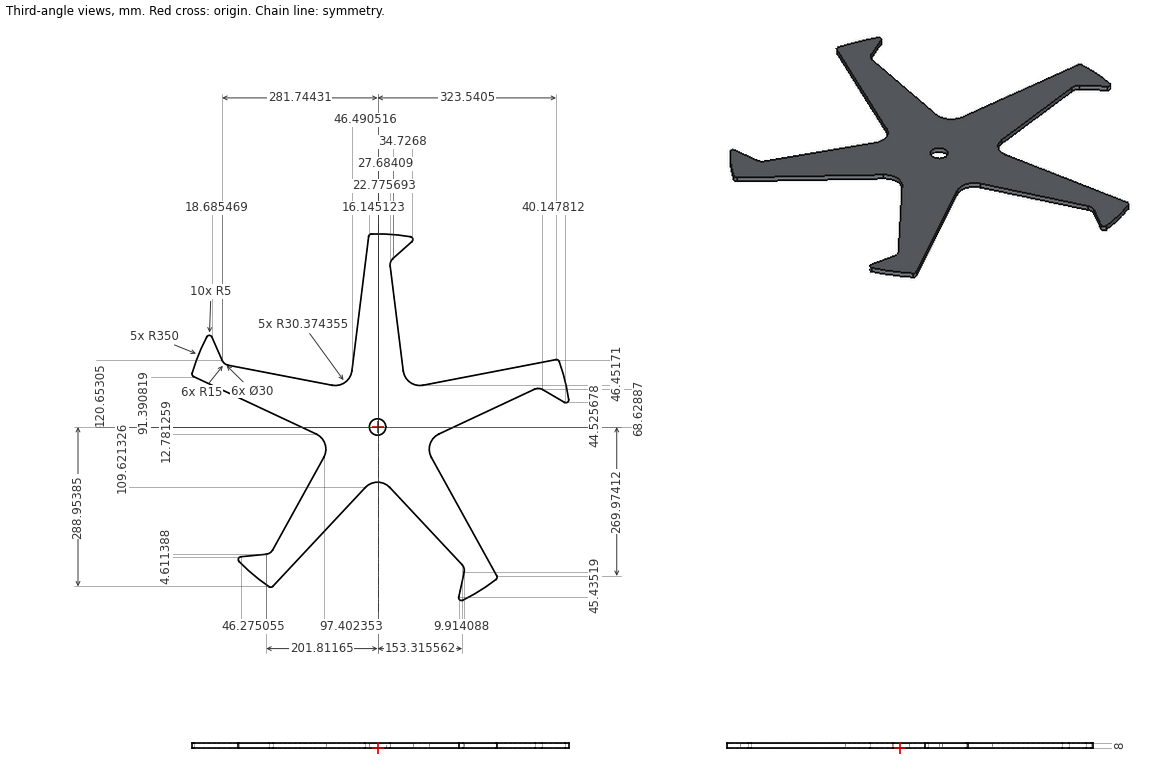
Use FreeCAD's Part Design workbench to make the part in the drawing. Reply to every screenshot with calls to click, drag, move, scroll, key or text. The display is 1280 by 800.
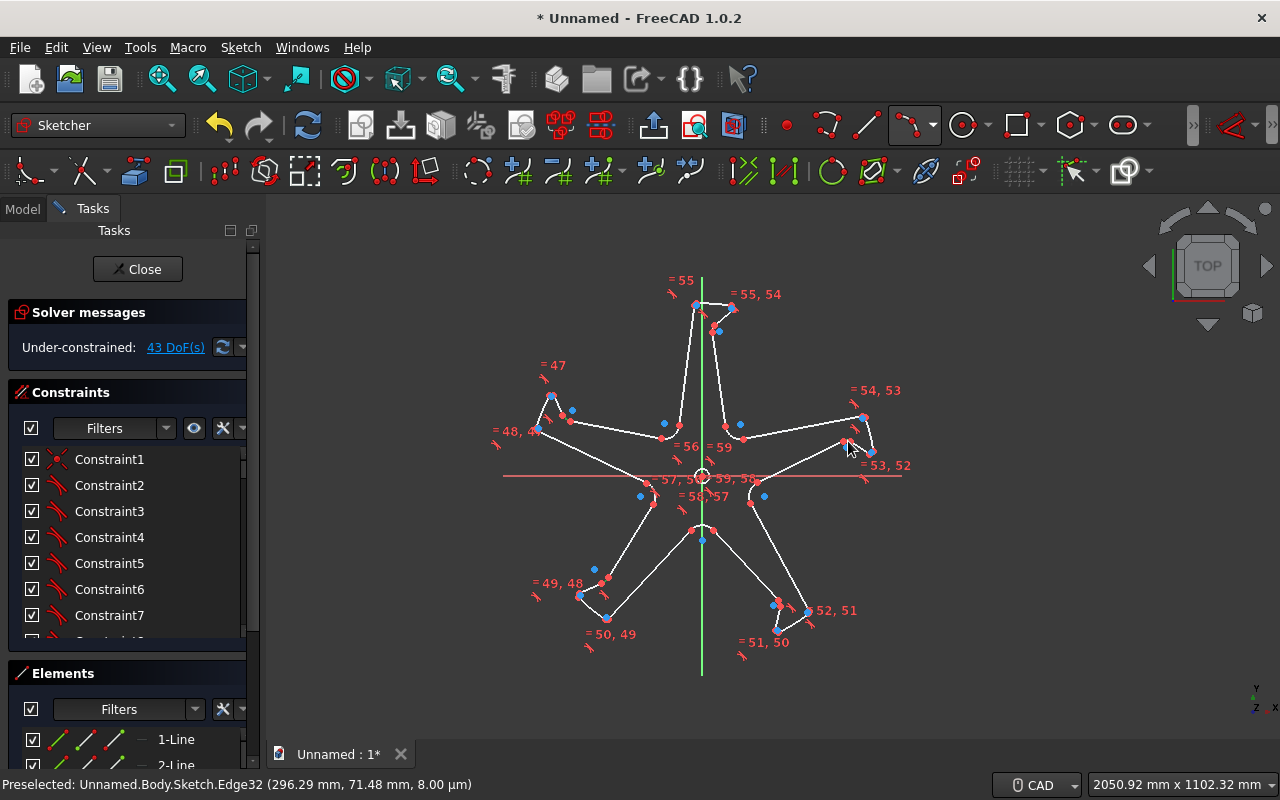
scroll(713, 327, up, 10)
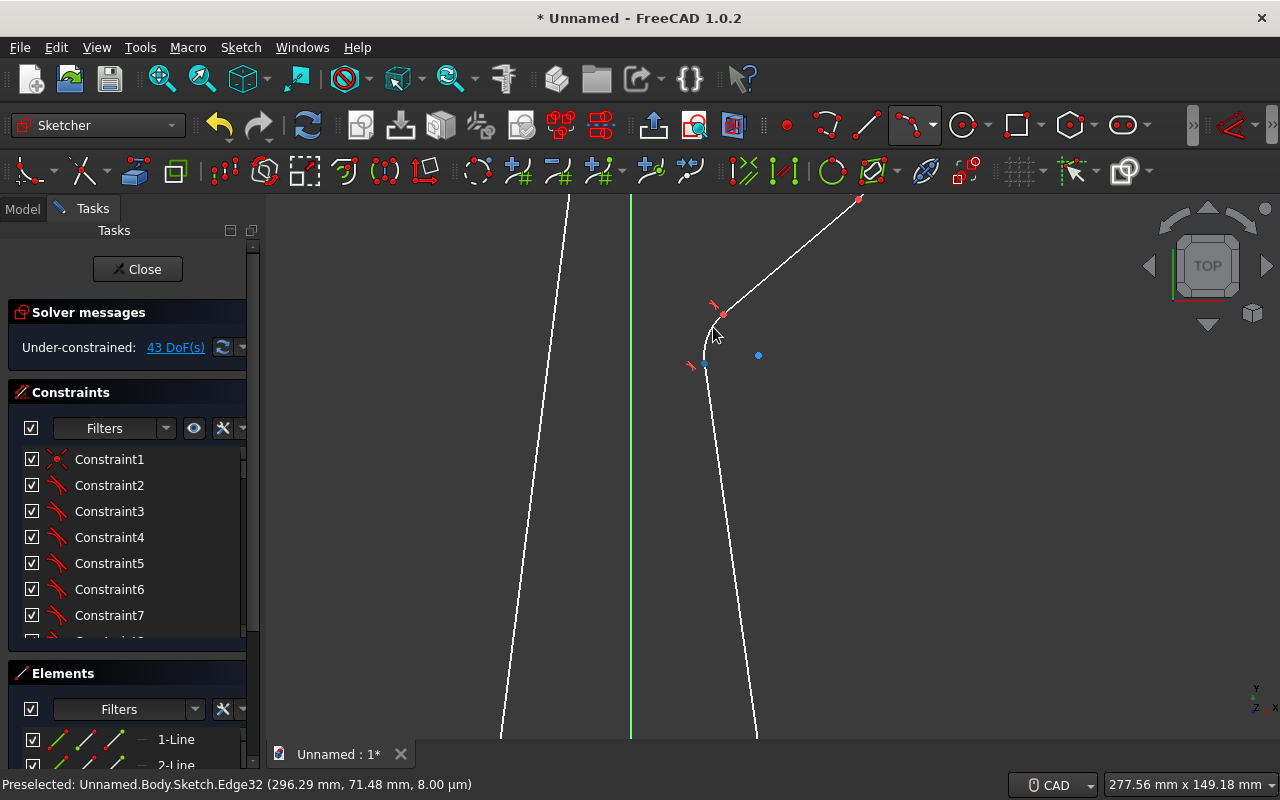
click(713, 327)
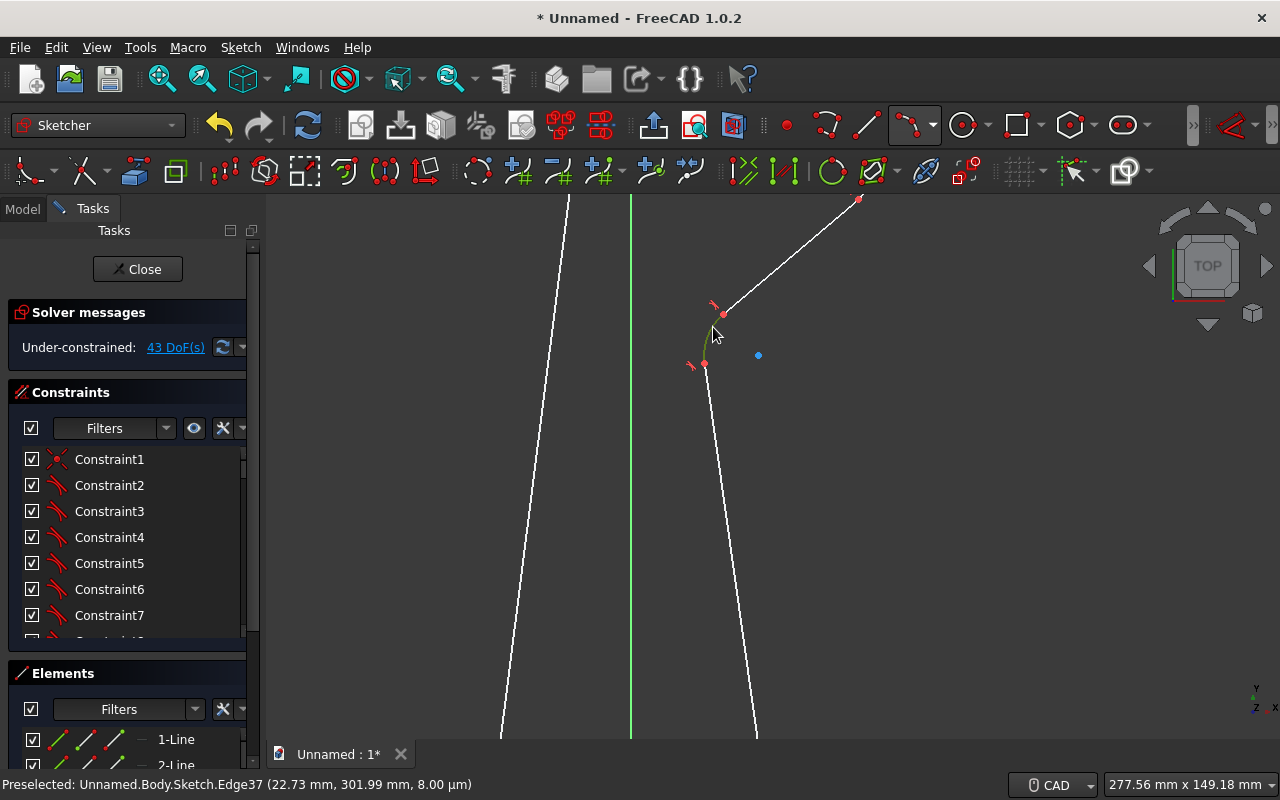
key(e)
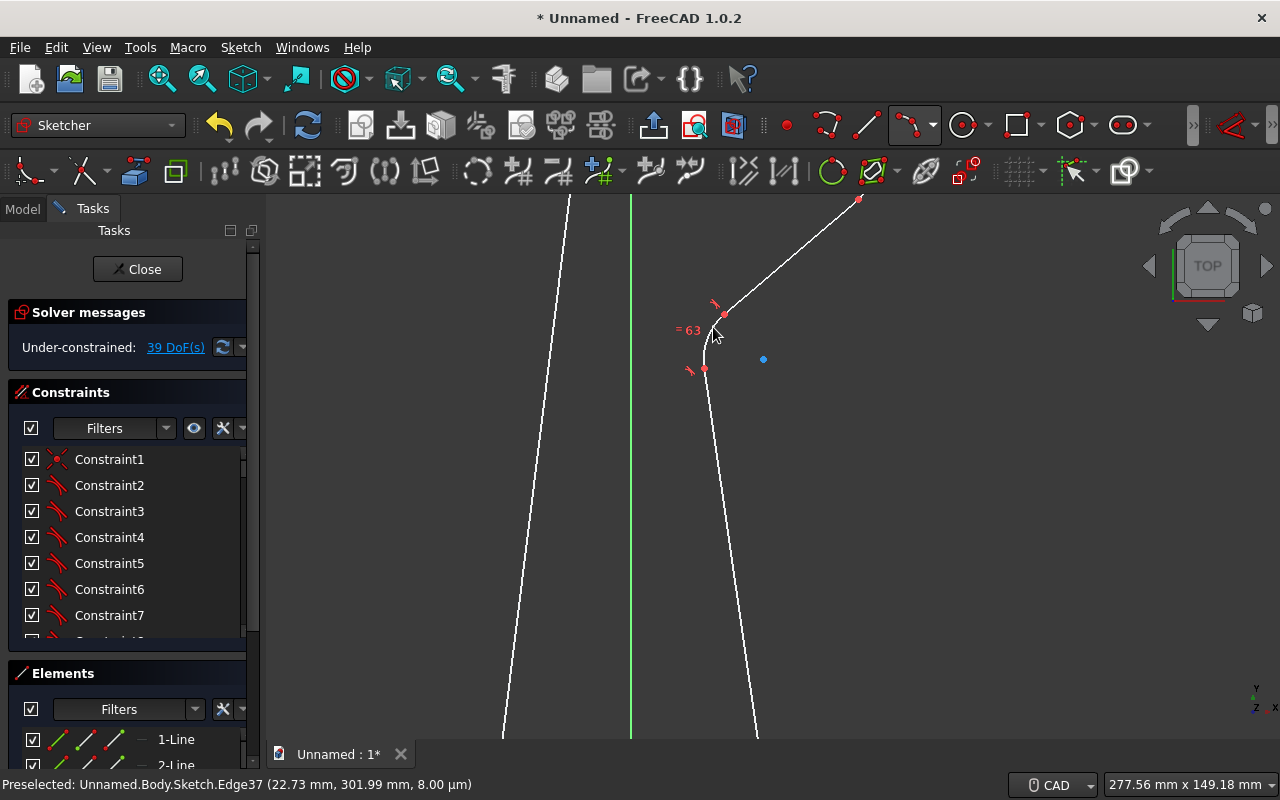
scroll(713, 326, down, 10)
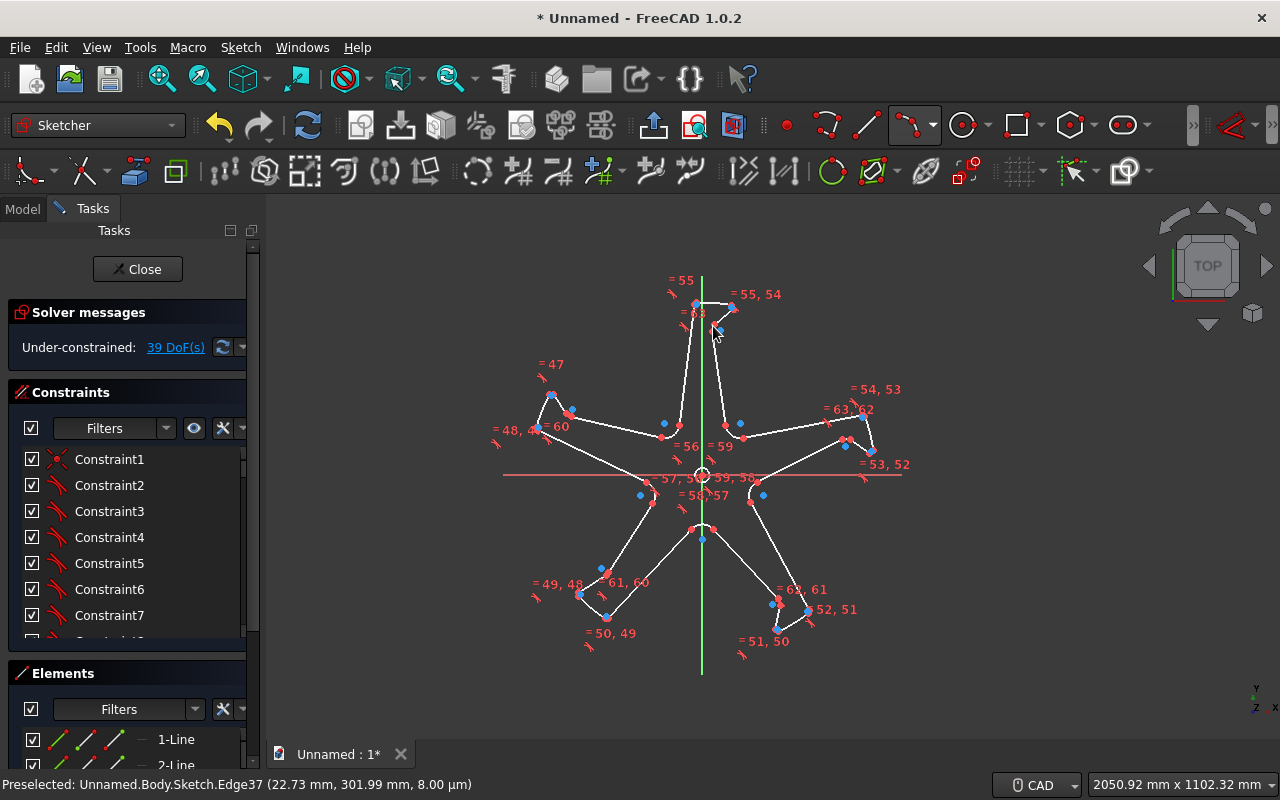
scroll(545, 404, up, 2)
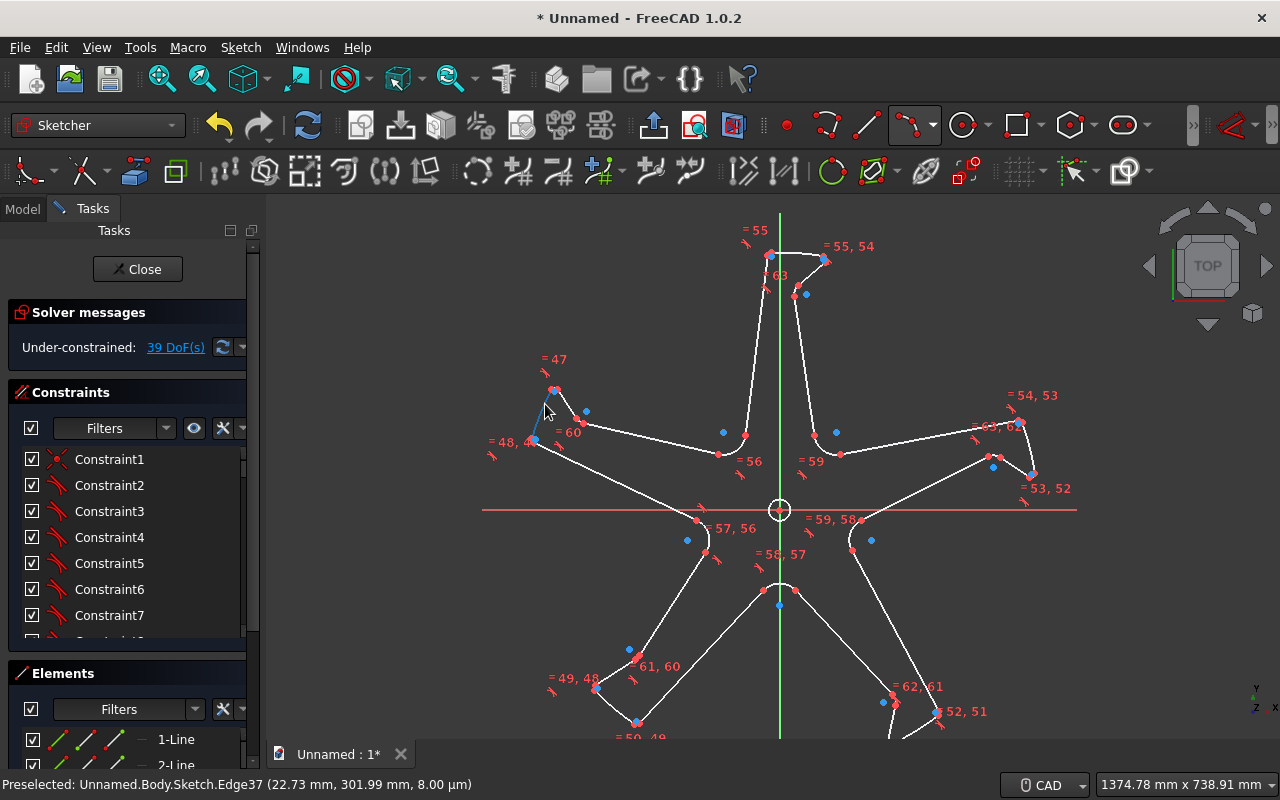
click(545, 404)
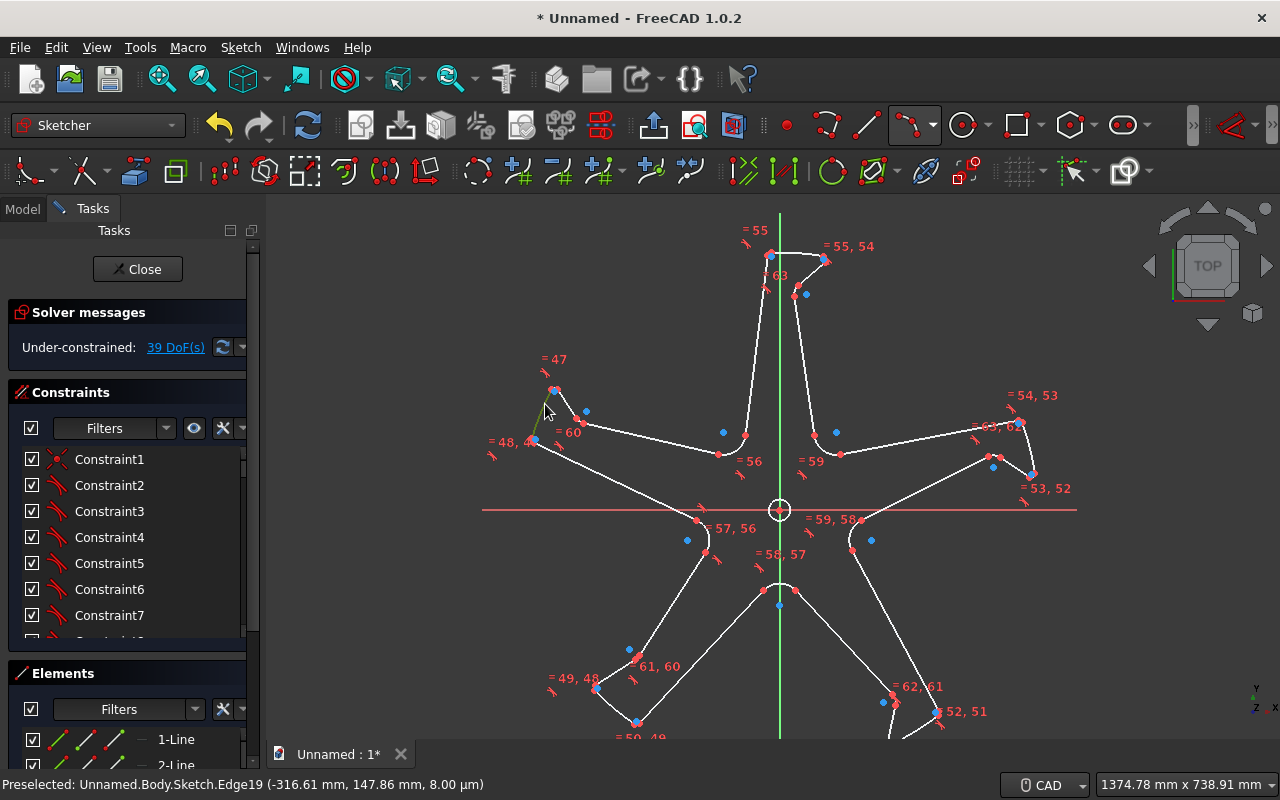
click(606, 701)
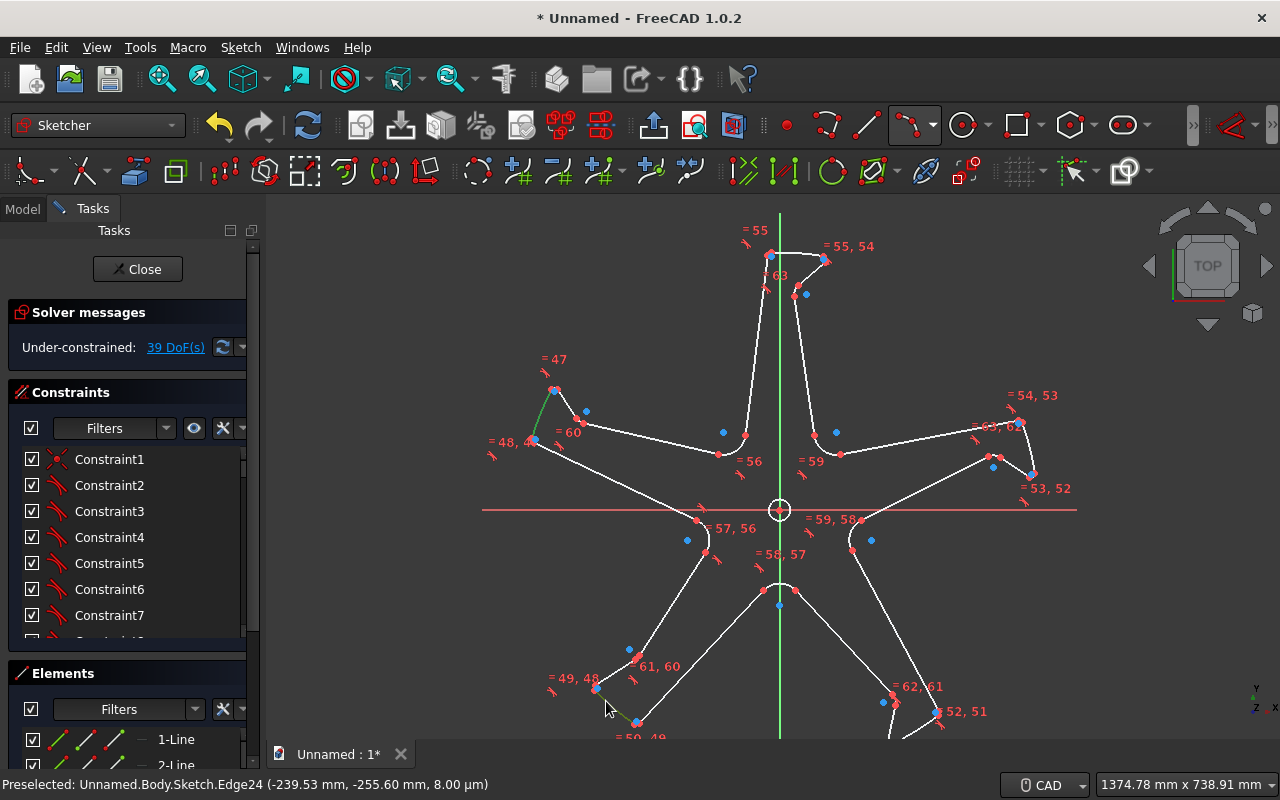
scroll(544, 405, down, 2)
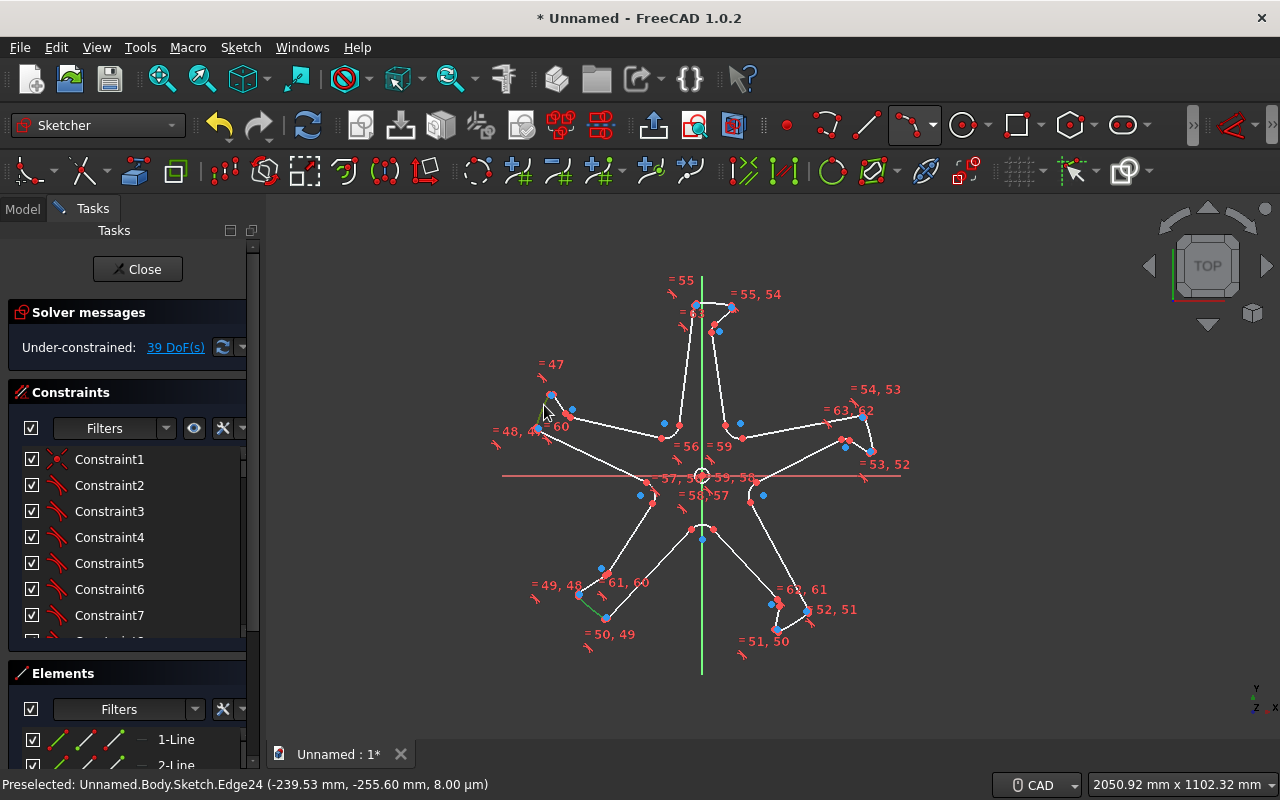
scroll(788, 627, up, 2)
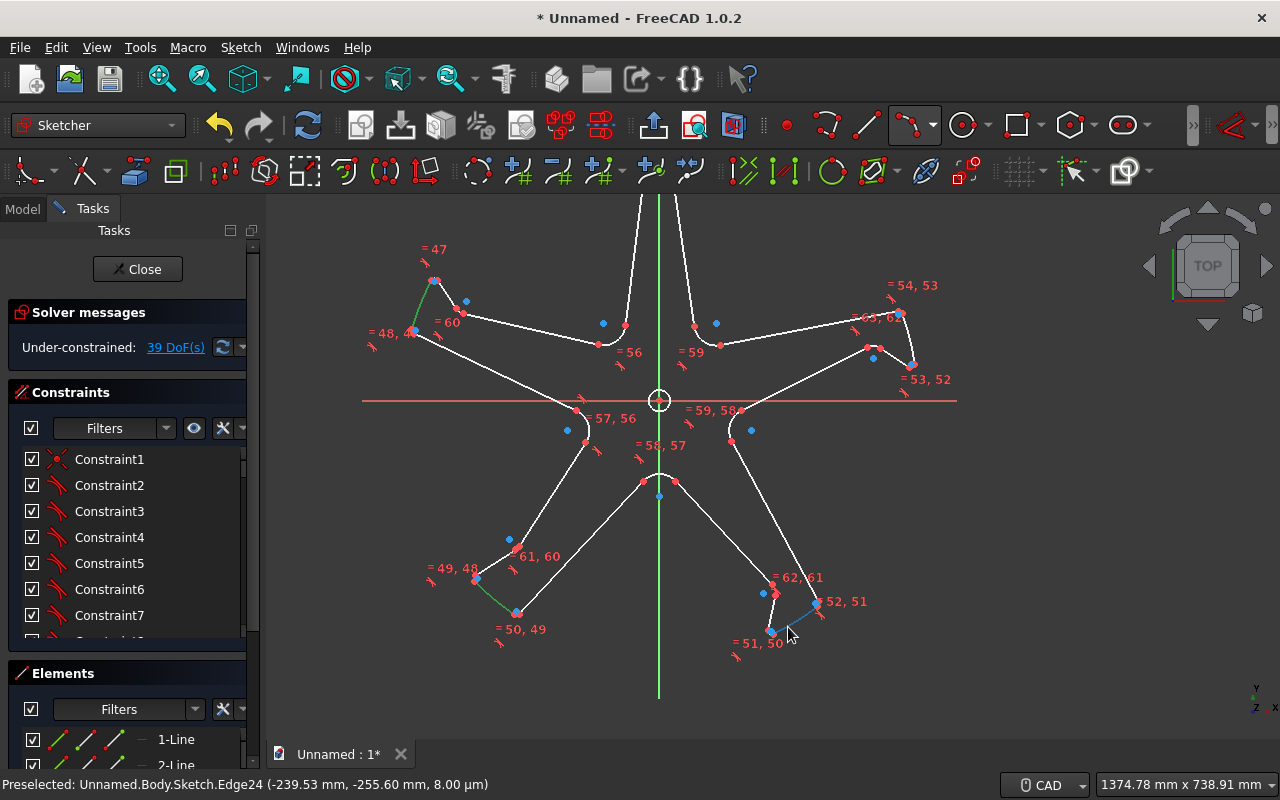
click(787, 627)